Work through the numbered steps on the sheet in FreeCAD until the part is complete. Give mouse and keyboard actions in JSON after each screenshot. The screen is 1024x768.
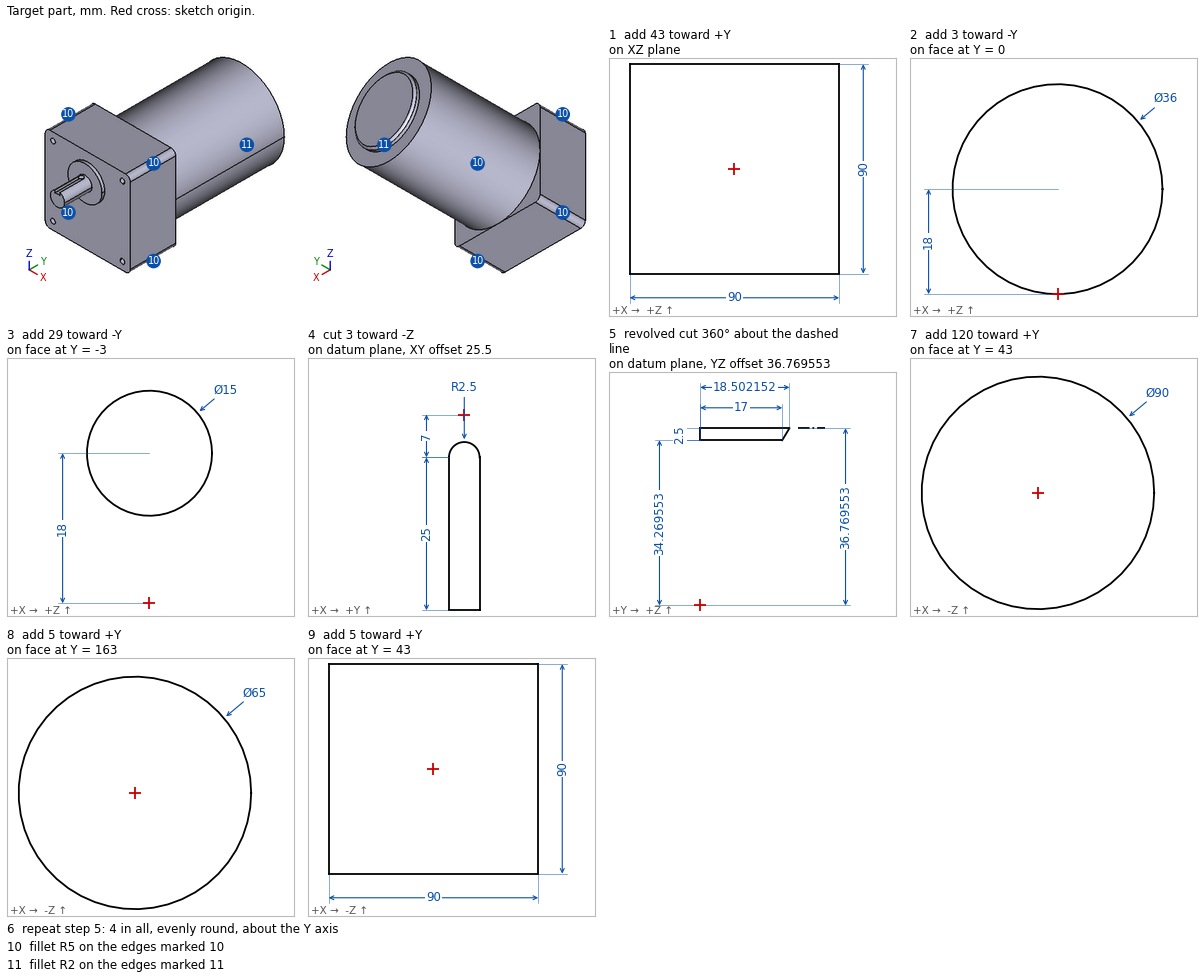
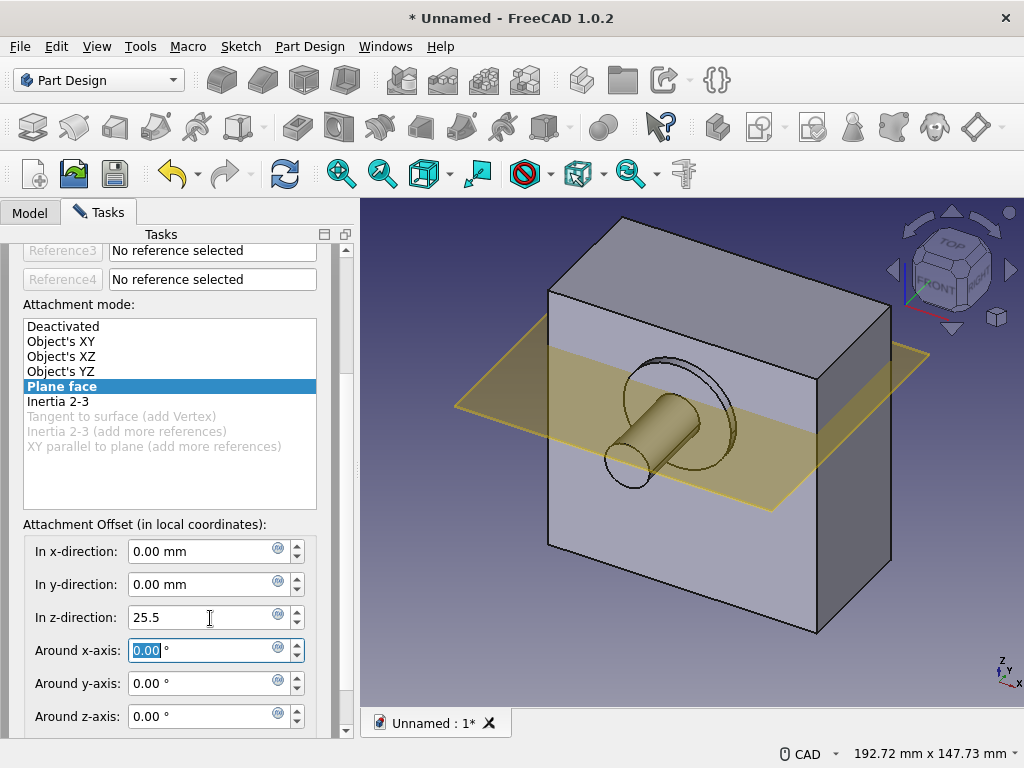
{"action": "scroll", "coordinate": [346, 491], "scroll_direction": "up", "scroll_amount": 4}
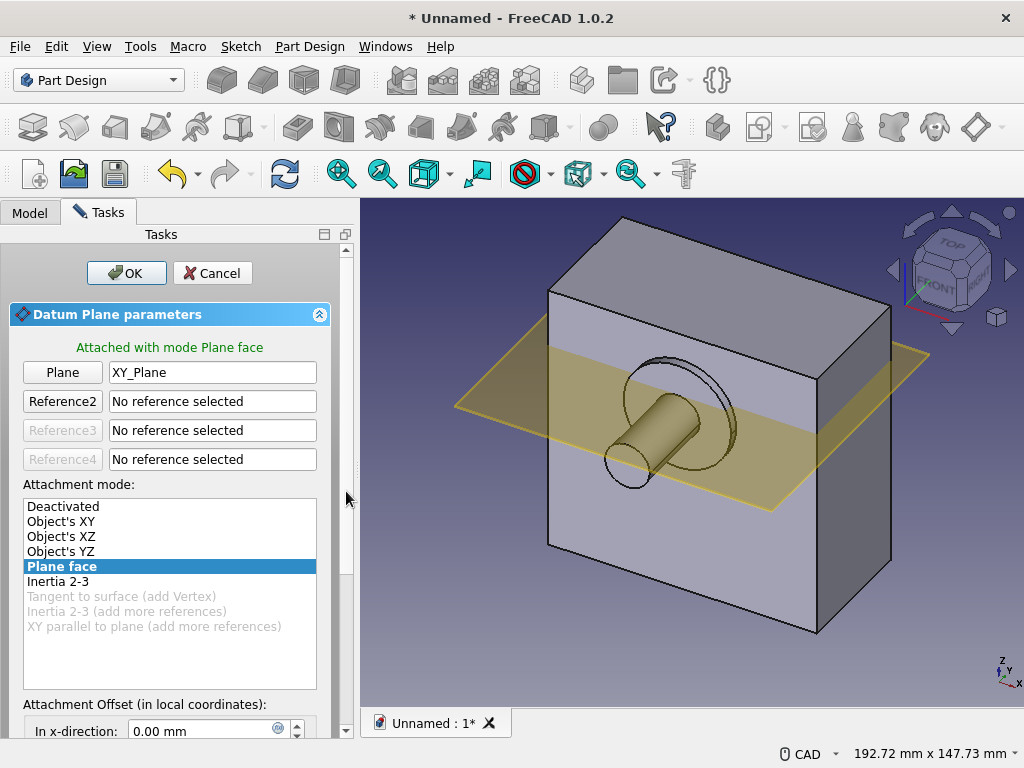
{"action": "left_click", "coordinate": [127, 273]}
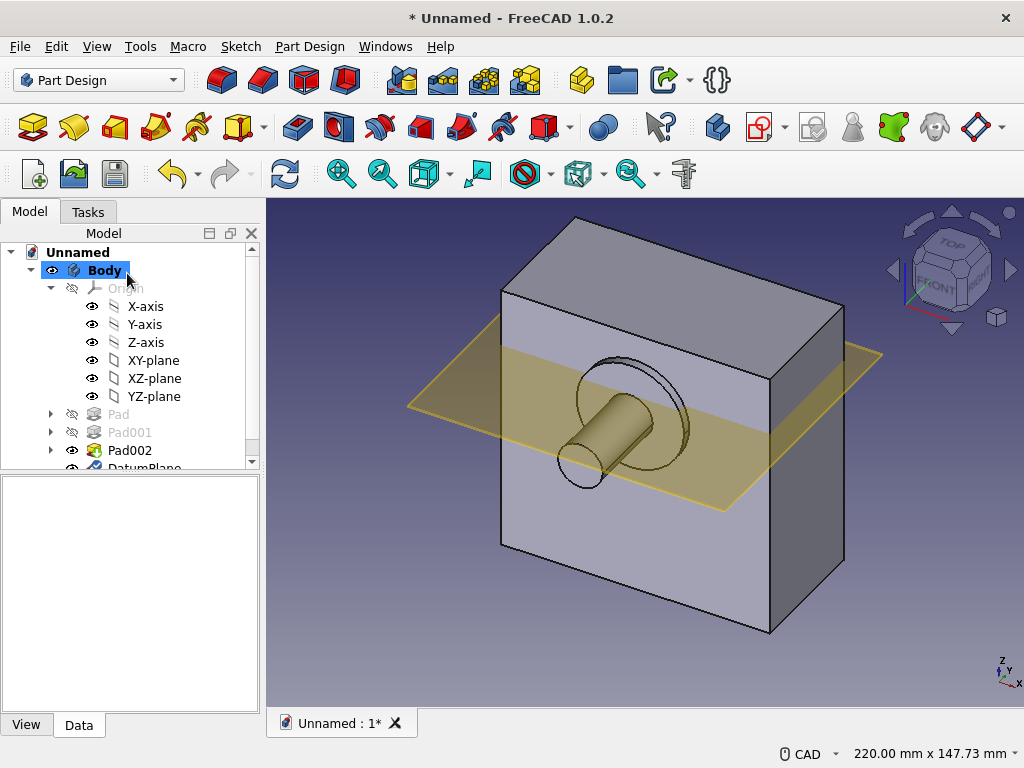
{"action": "left_click", "coordinate": [117, 468]}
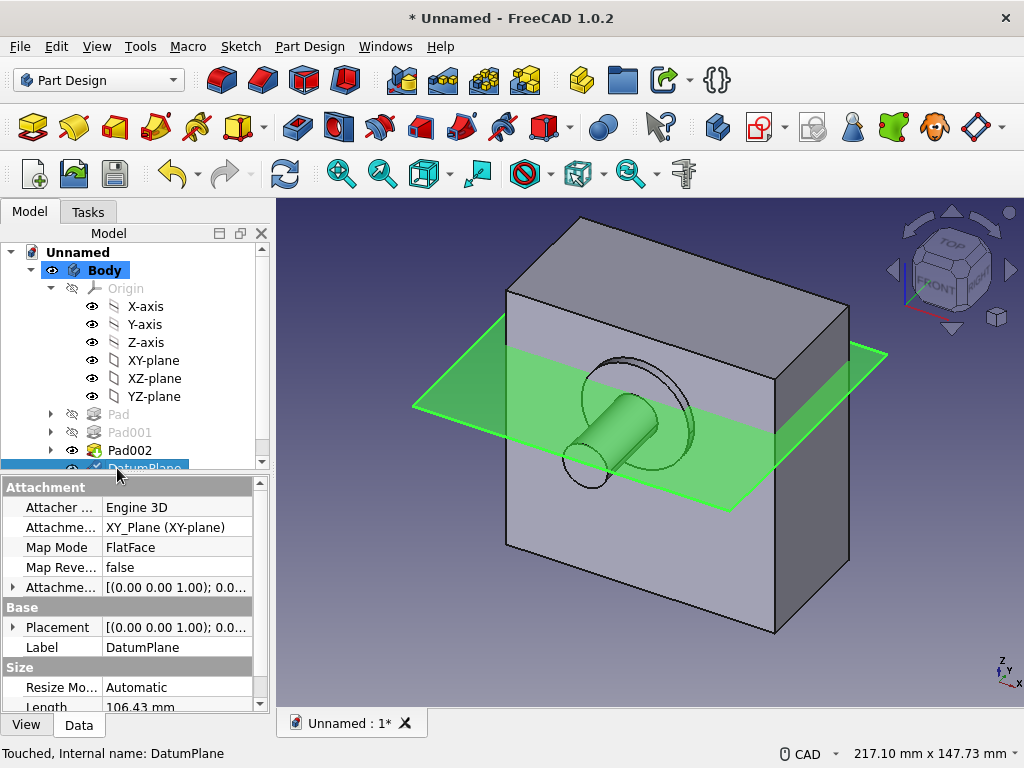
{"action": "left_click", "coordinate": [758, 128]}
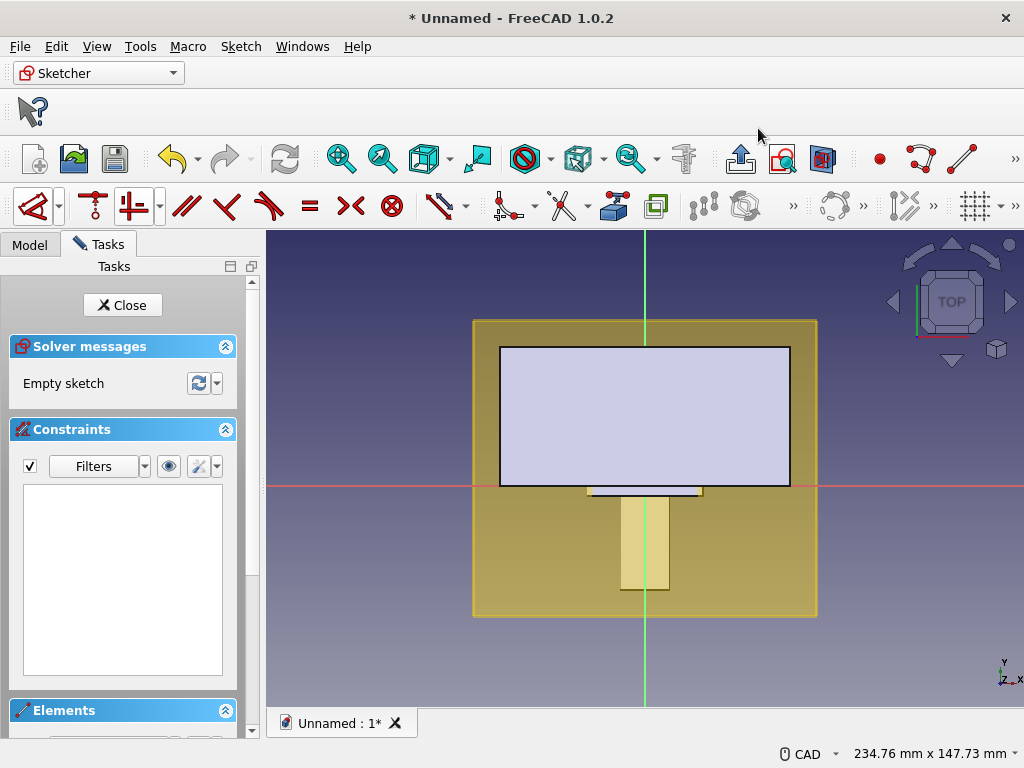
{"action": "left_click", "coordinate": [823, 160]}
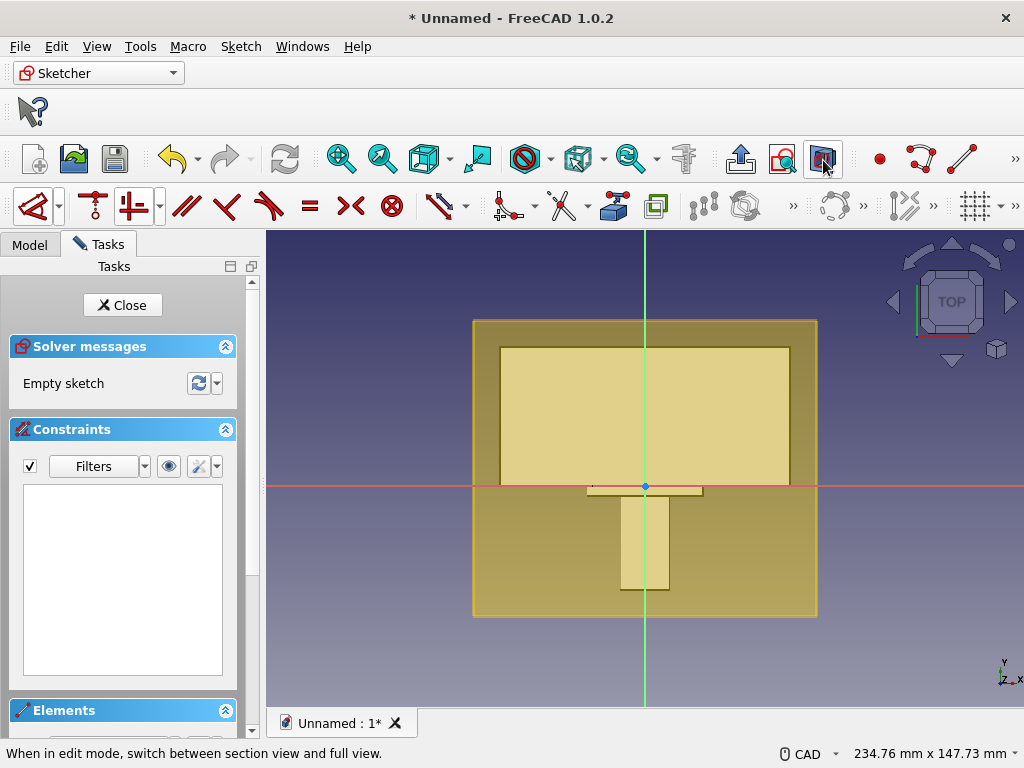
{"action": "scroll", "coordinate": [685, 578], "scroll_direction": "up", "scroll_amount": 5}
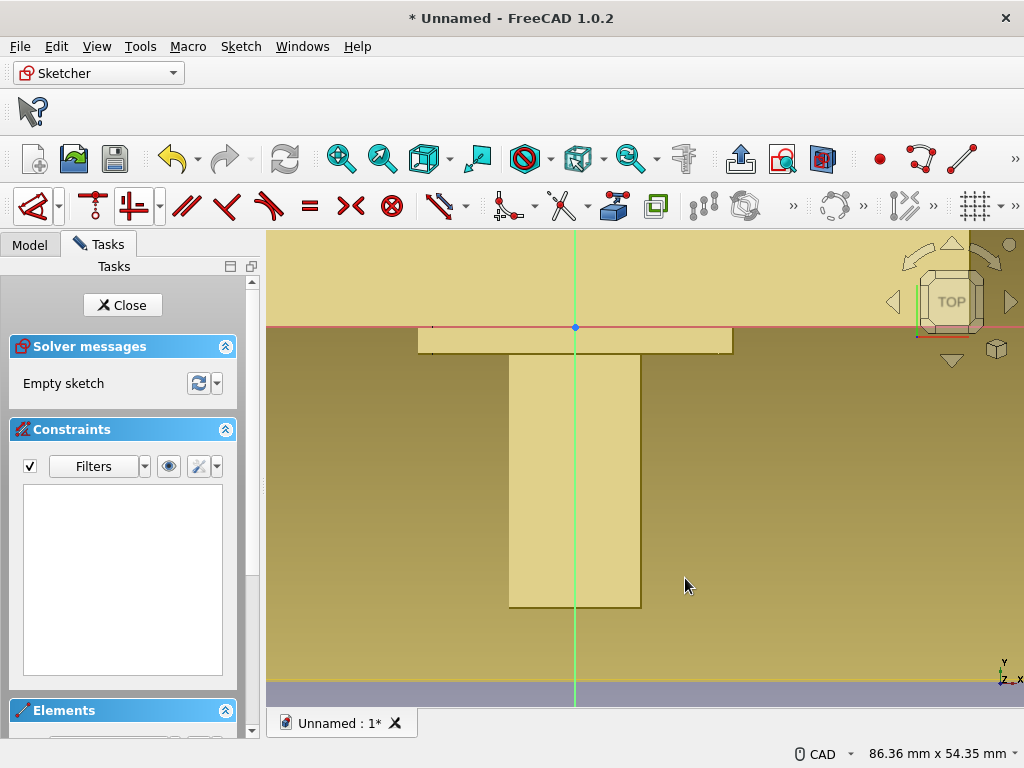
{"action": "left_click", "coordinate": [921, 160]}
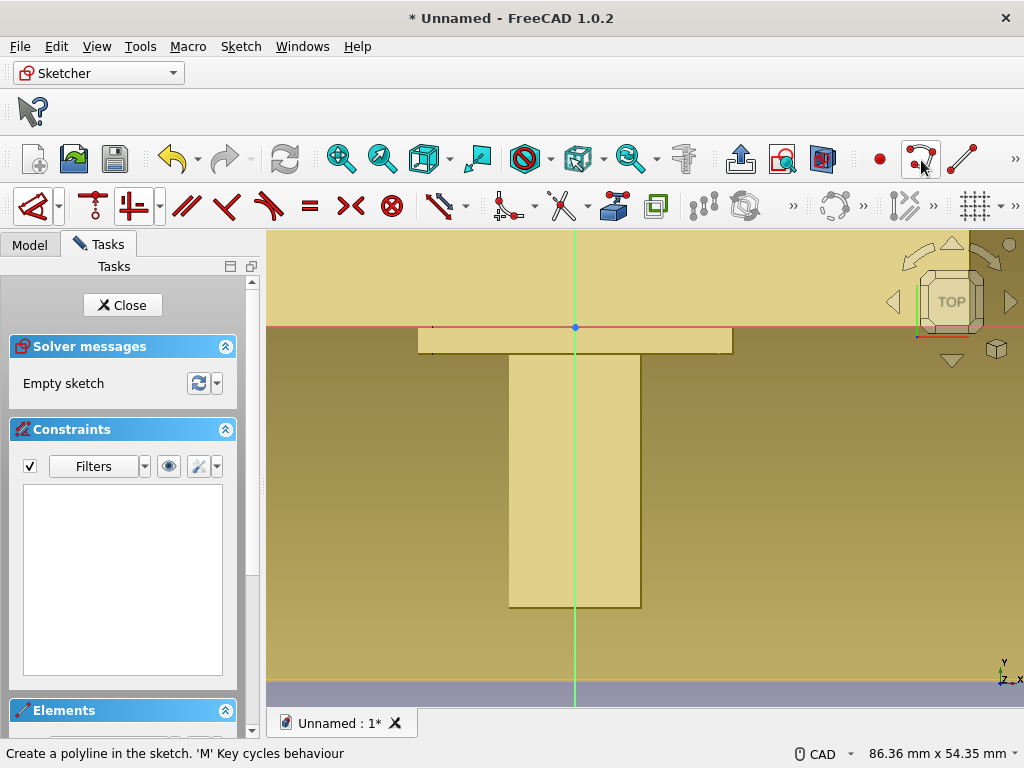
{"action": "left_click", "coordinate": [553, 389]}
{"action": "left_click", "coordinate": [553, 608]}
{"action": "left_click", "coordinate": [597, 608]}
{"action": "left_click", "coordinate": [597, 389]}
{"action": "right_click", "coordinate": [597, 389]}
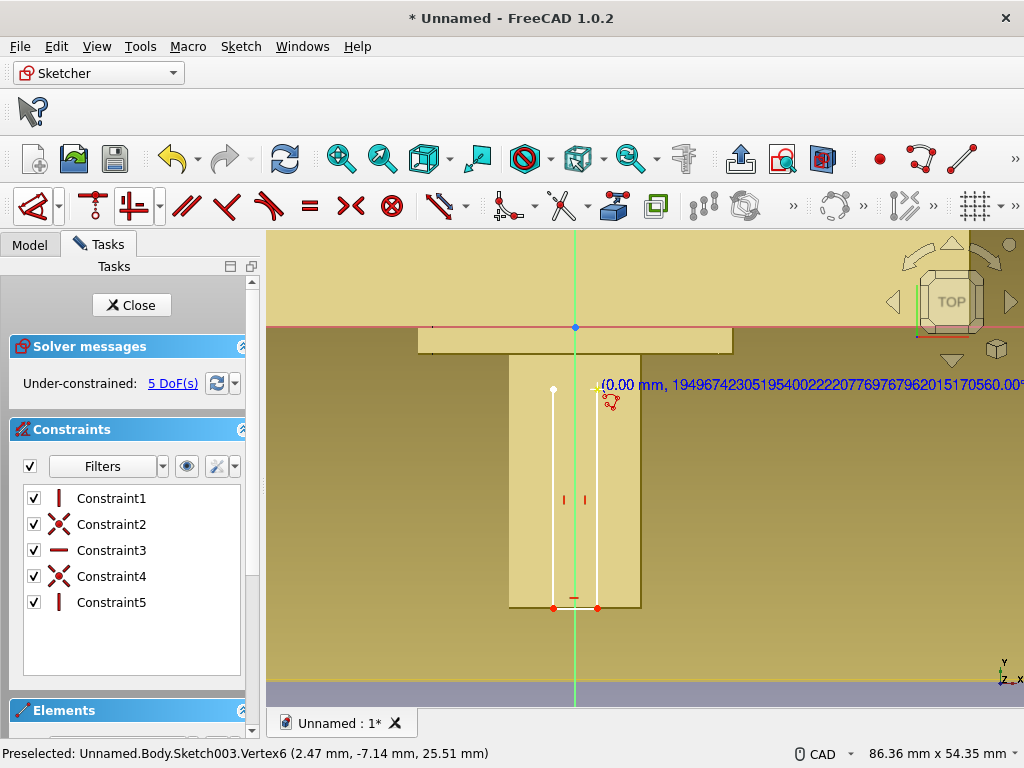
{"action": "key", "text": "g 3 a"}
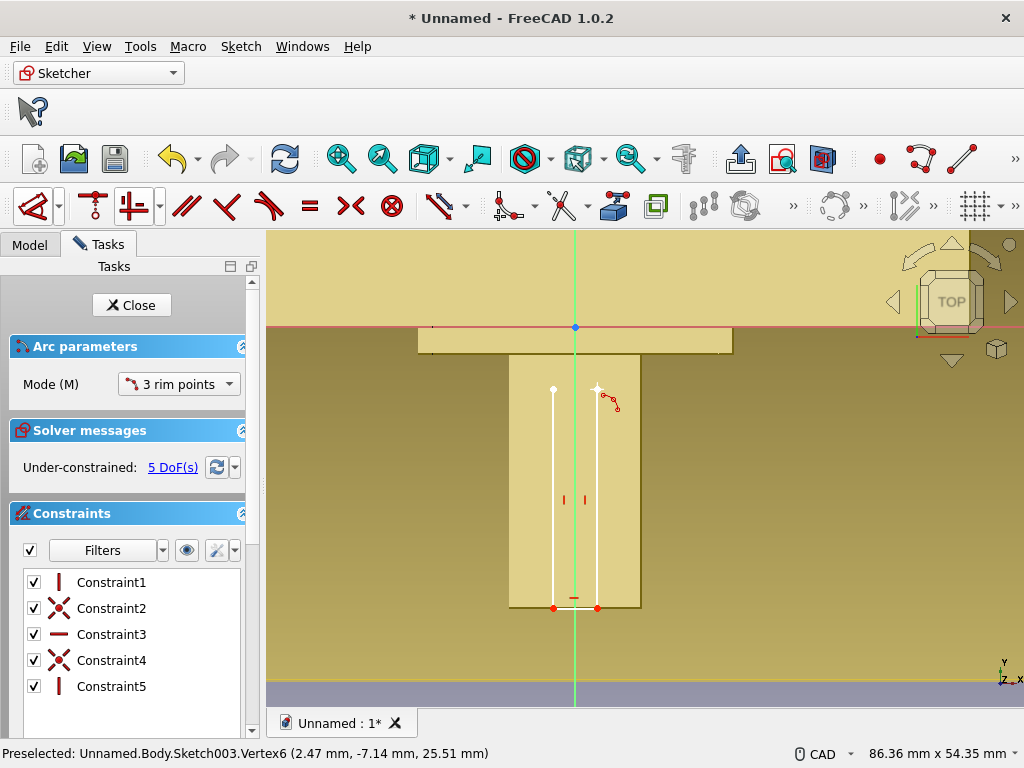
{"action": "left_click", "coordinate": [597, 390]}
{"action": "left_click", "coordinate": [553, 390]}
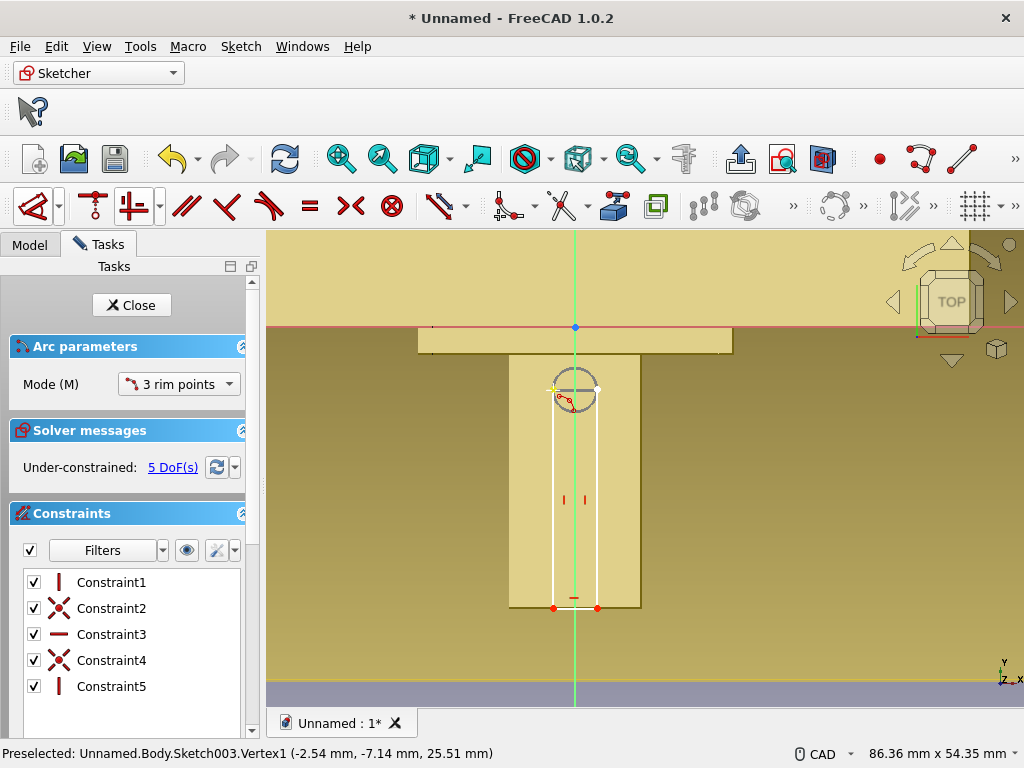
{"action": "scroll", "coordinate": [588, 371], "scroll_direction": "up", "scroll_amount": 2}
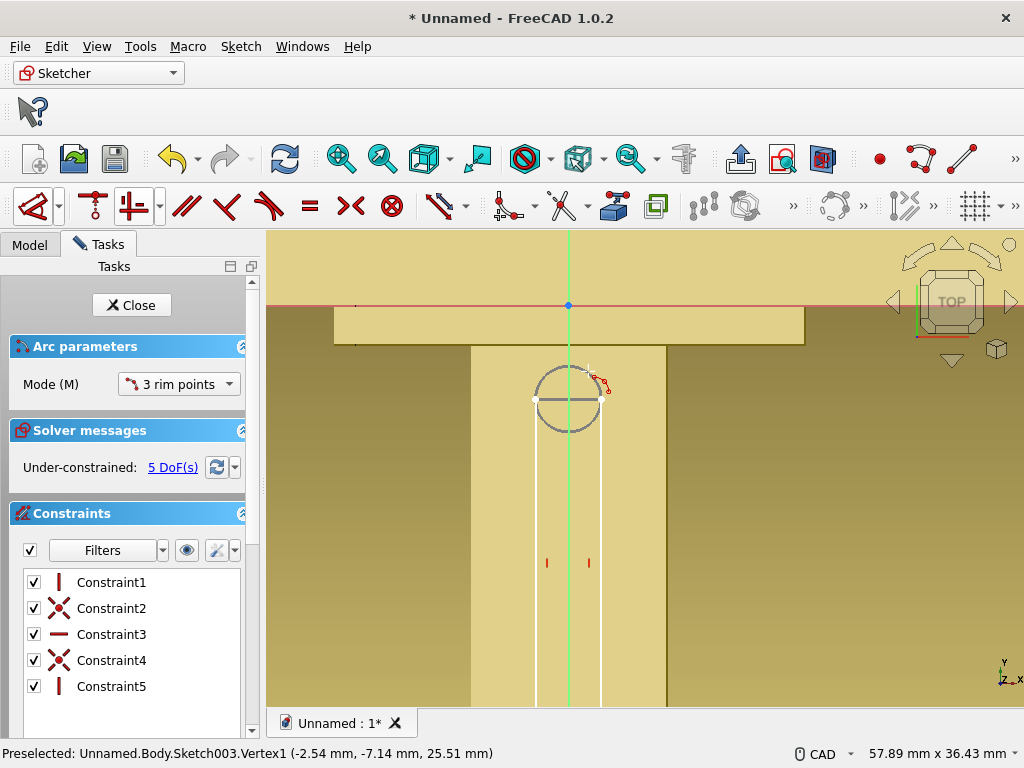
{"action": "left_click", "coordinate": [588, 371]}
{"action": "key", "text": "Escape"}